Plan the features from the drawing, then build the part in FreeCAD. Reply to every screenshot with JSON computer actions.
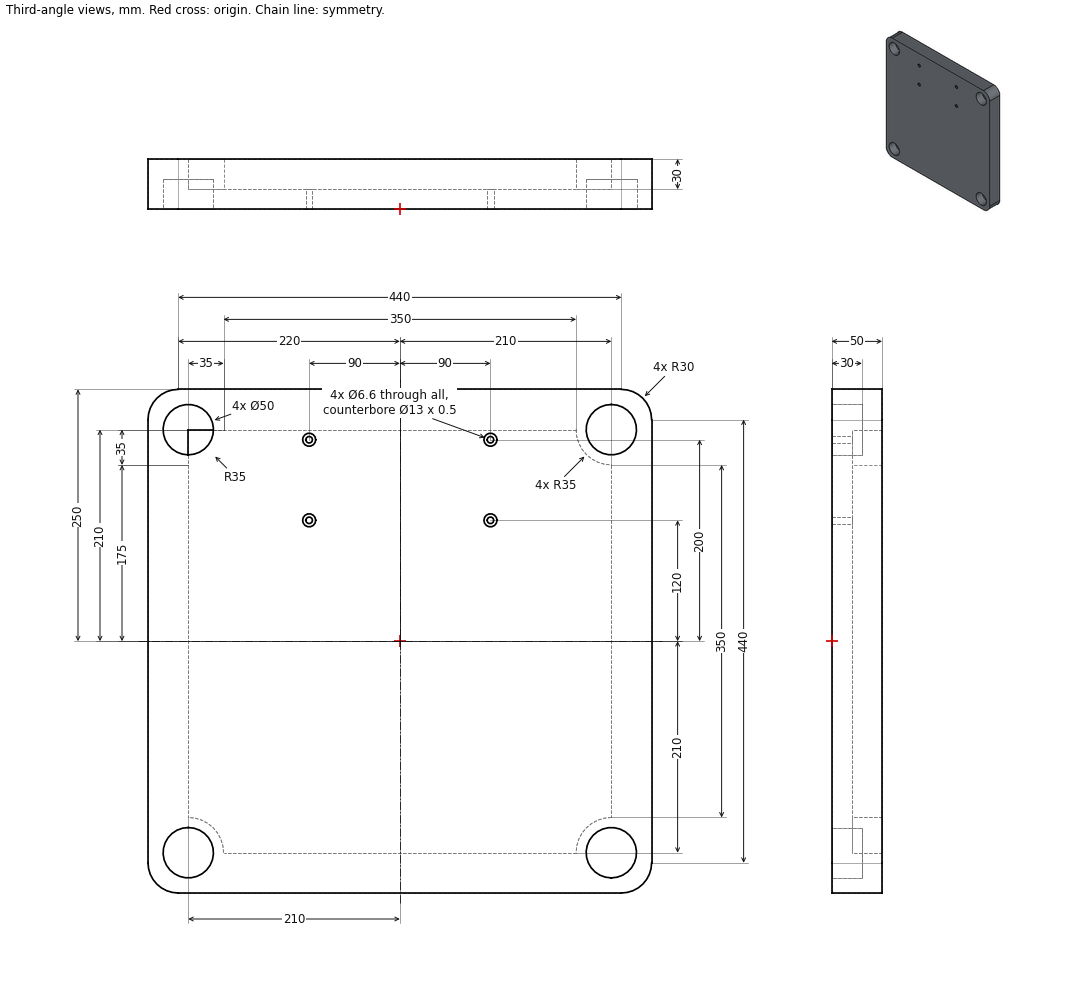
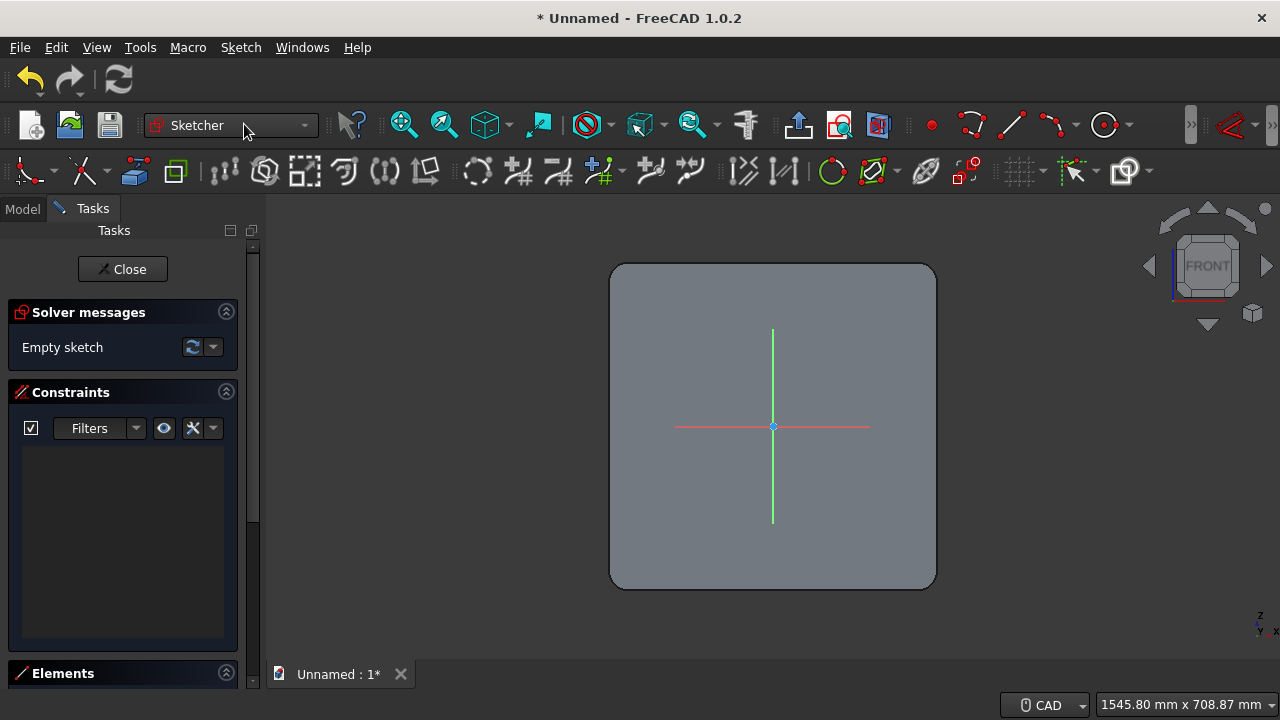
{"action": "key", "text": "g c"}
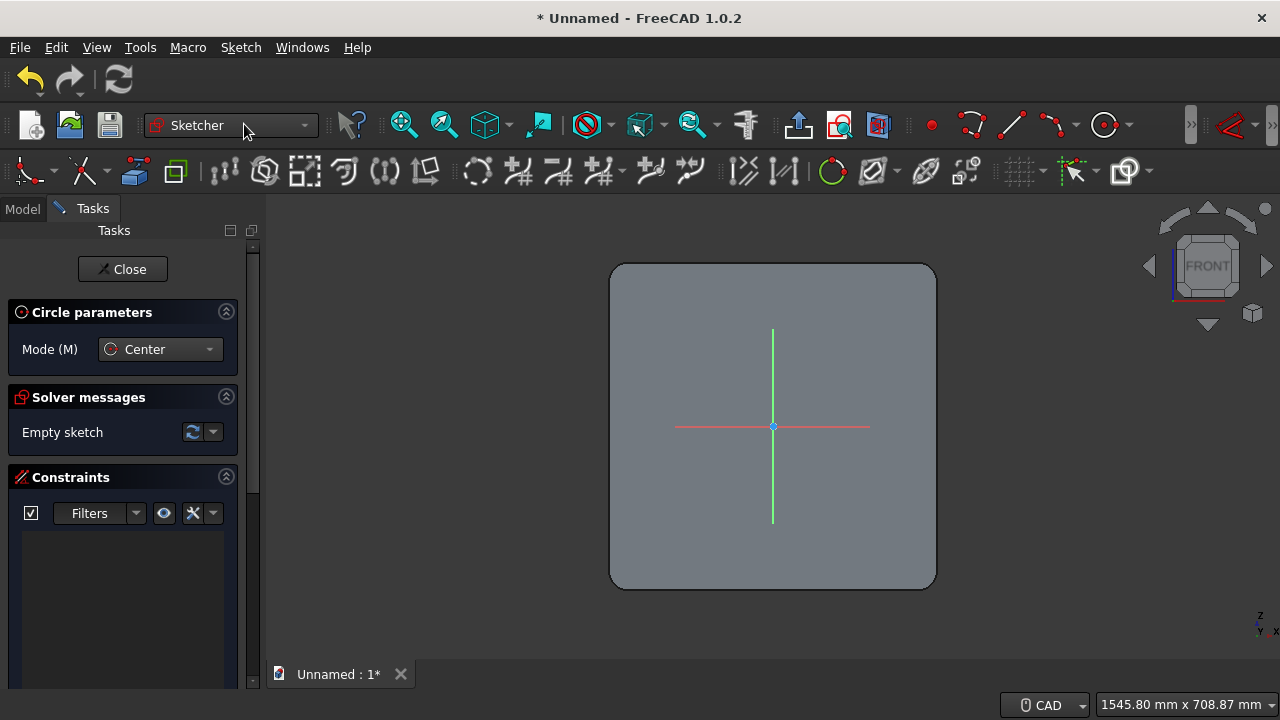
{"action": "scroll", "coordinate": [635, 289], "scroll_direction": "up", "scroll_amount": 2}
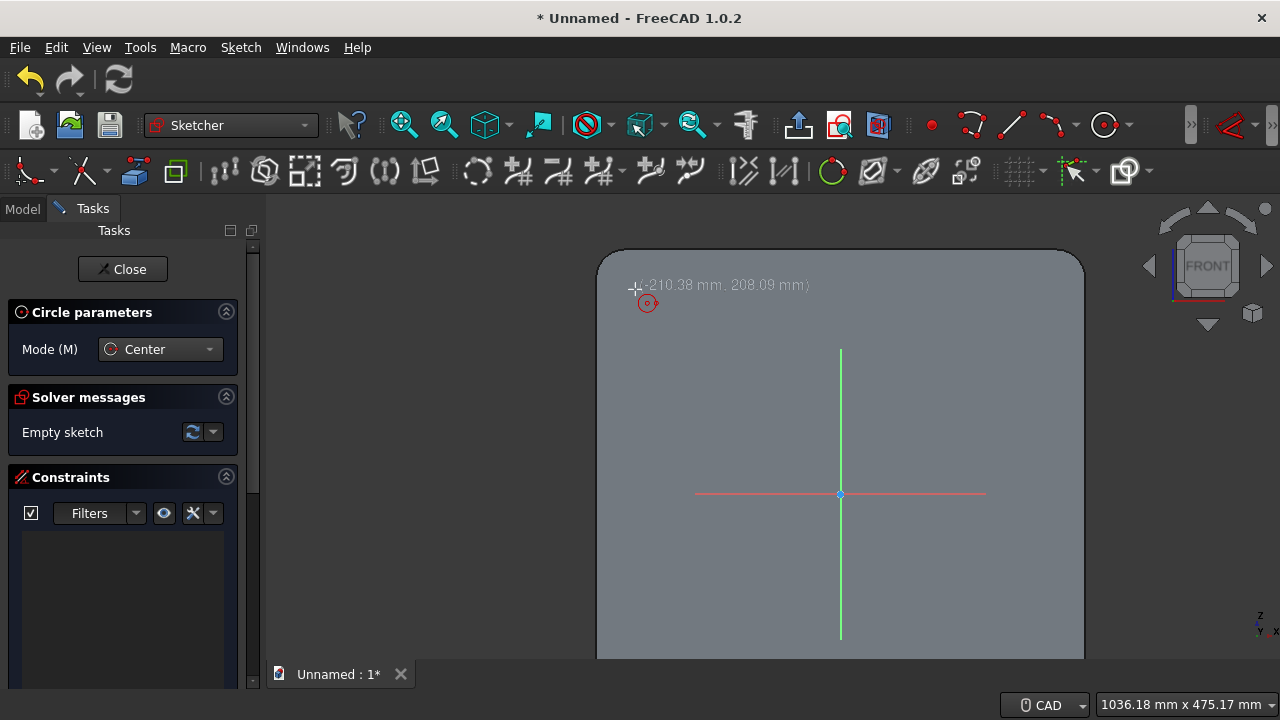
{"action": "left_click", "coordinate": [635, 289]}
{"action": "left_click", "coordinate": [652, 271]}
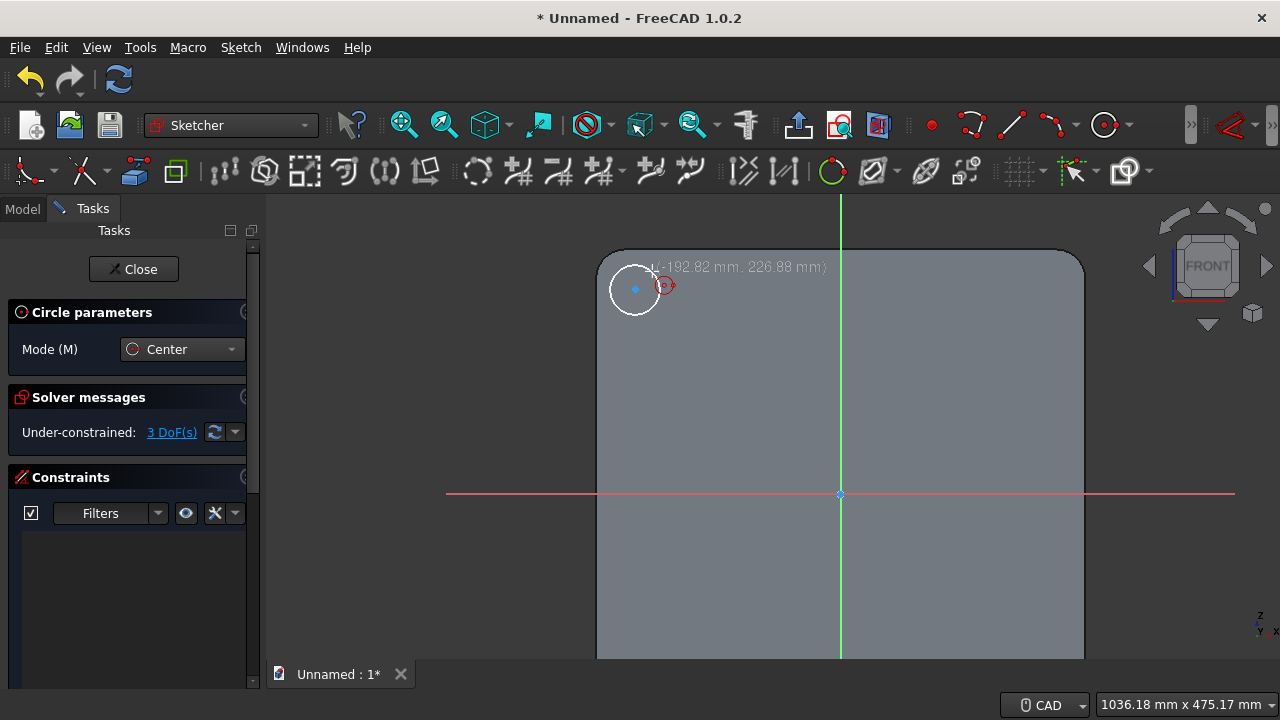
{"action": "left_click", "coordinate": [1046, 289]}
{"action": "left_click", "coordinate": [1063, 271]}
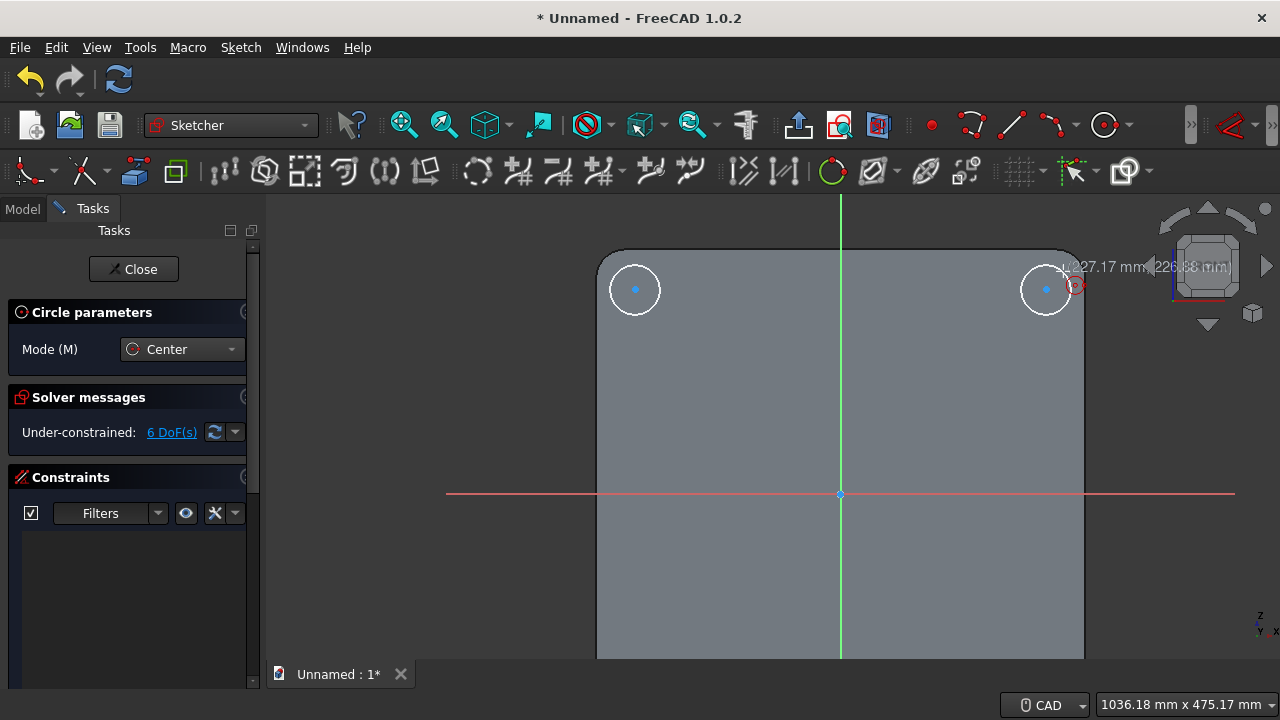
{"action": "scroll", "coordinate": [428, 289], "scroll_direction": "down", "scroll_amount": 2}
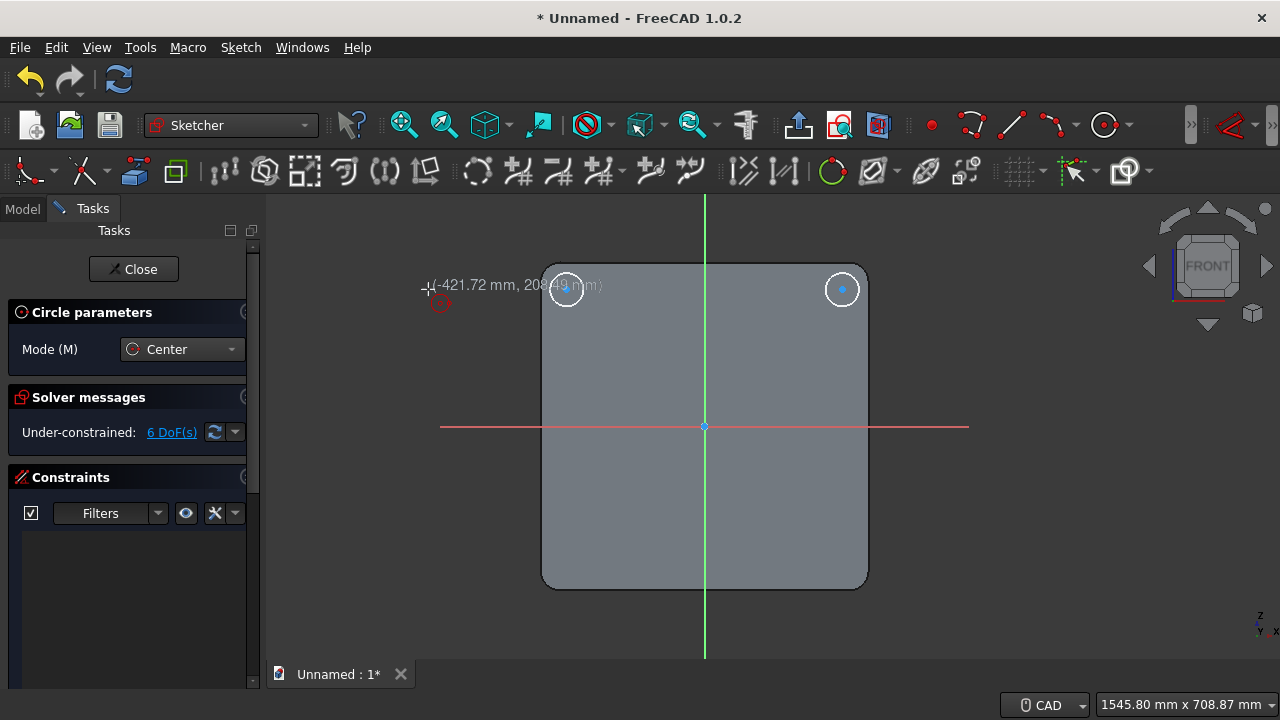
{"action": "scroll", "coordinate": [842, 564], "scroll_direction": "up", "scroll_amount": 2}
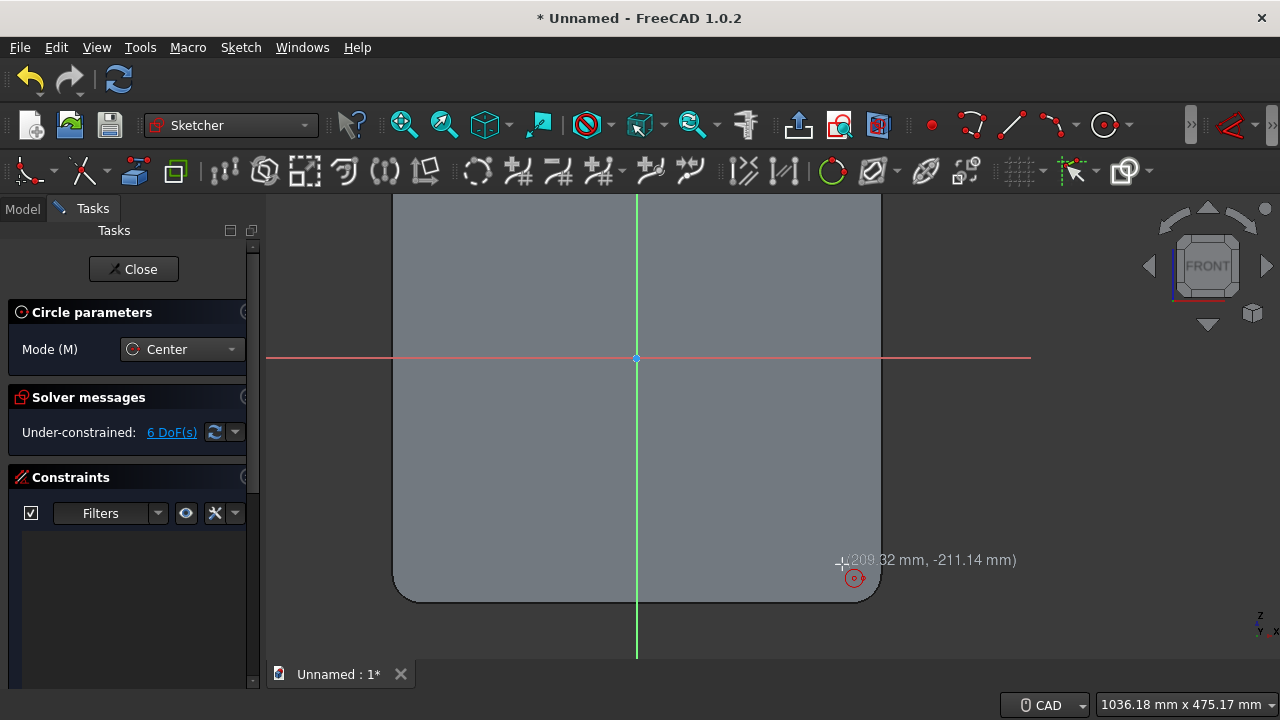
{"action": "left_click", "coordinate": [842, 564]}
{"action": "left_click", "coordinate": [860, 547]}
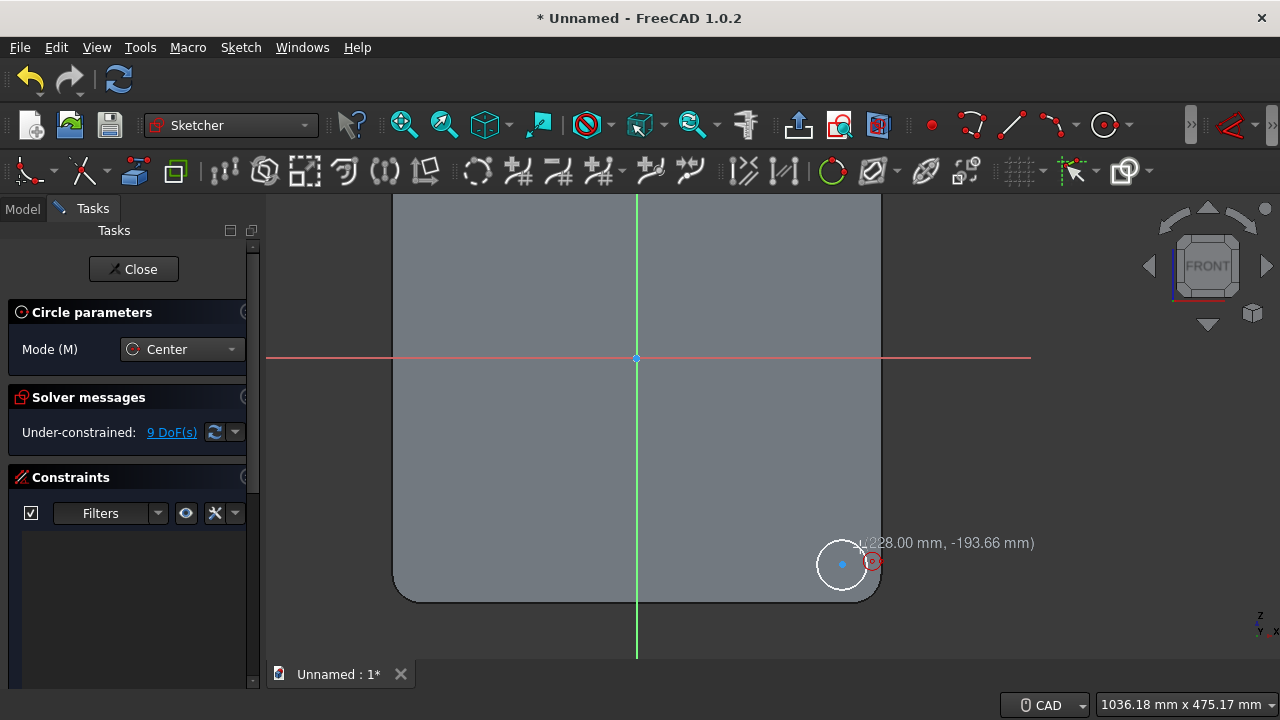
{"action": "left_click", "coordinate": [431, 564]}
{"action": "left_click", "coordinate": [449, 547]}
{"action": "key", "text": "Escape"}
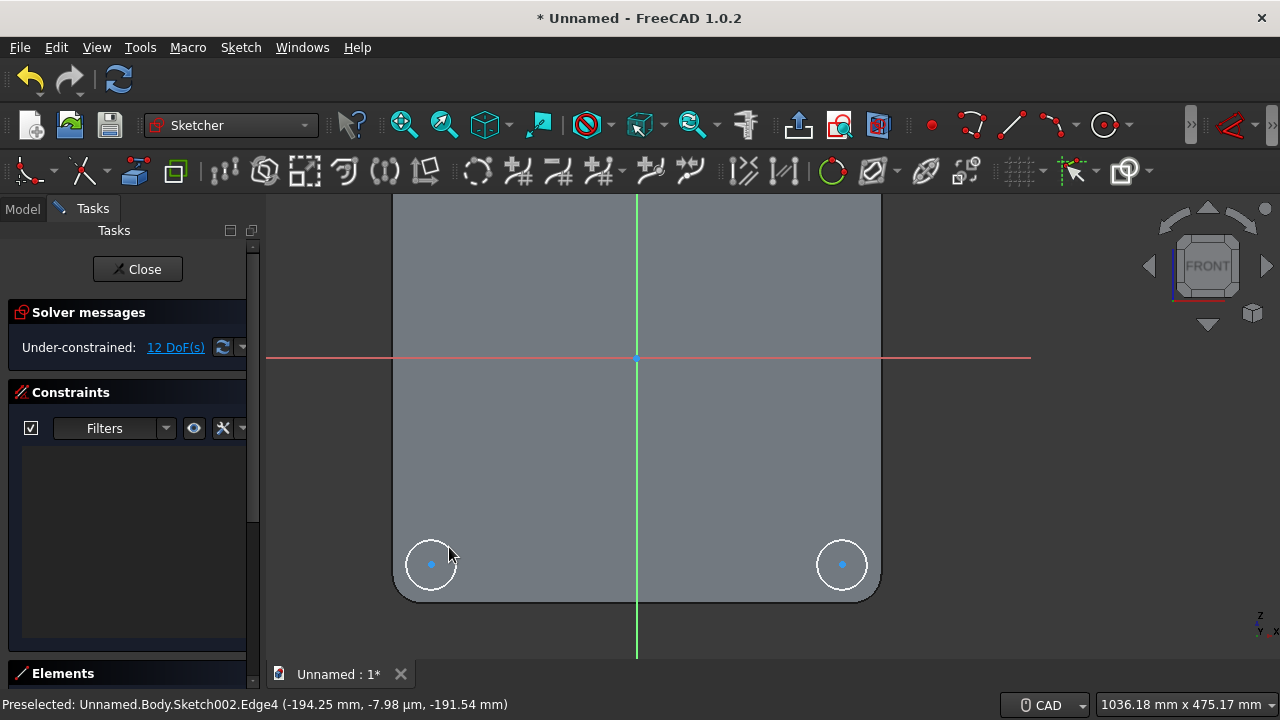
{"action": "scroll", "coordinate": [842, 565], "scroll_direction": "down", "scroll_amount": 2}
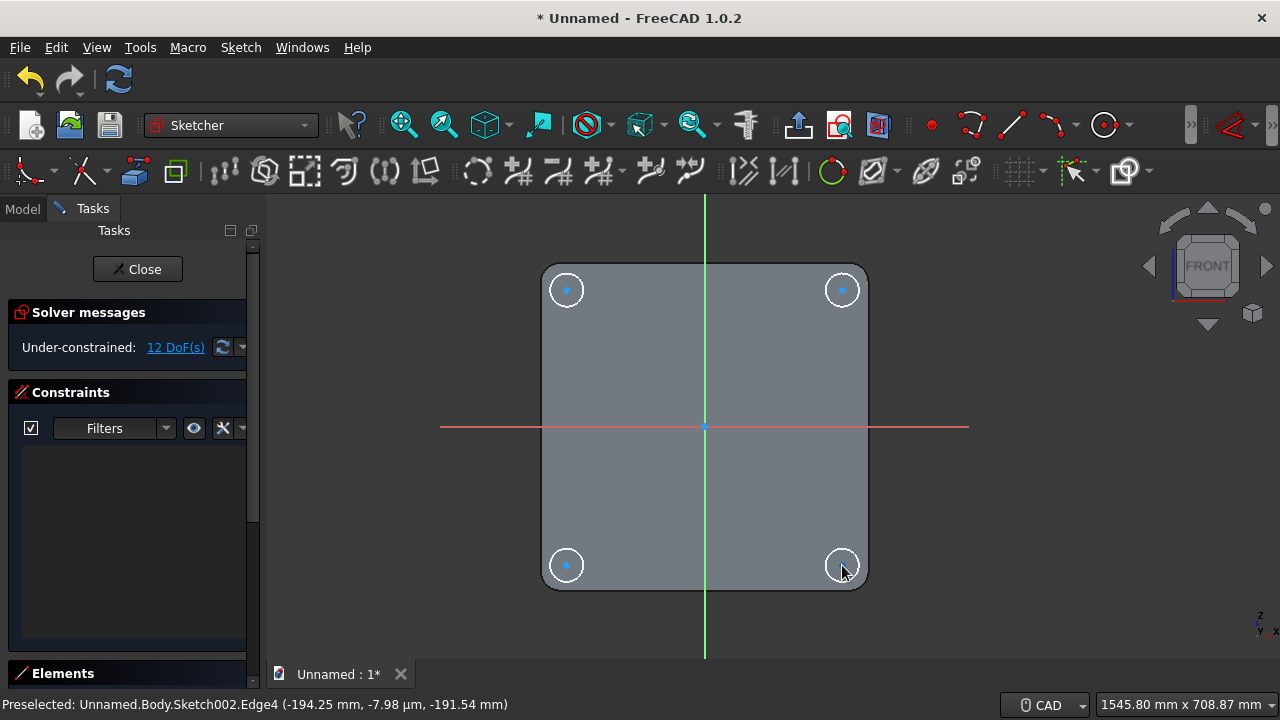
{"action": "left_click", "coordinate": [579, 278]}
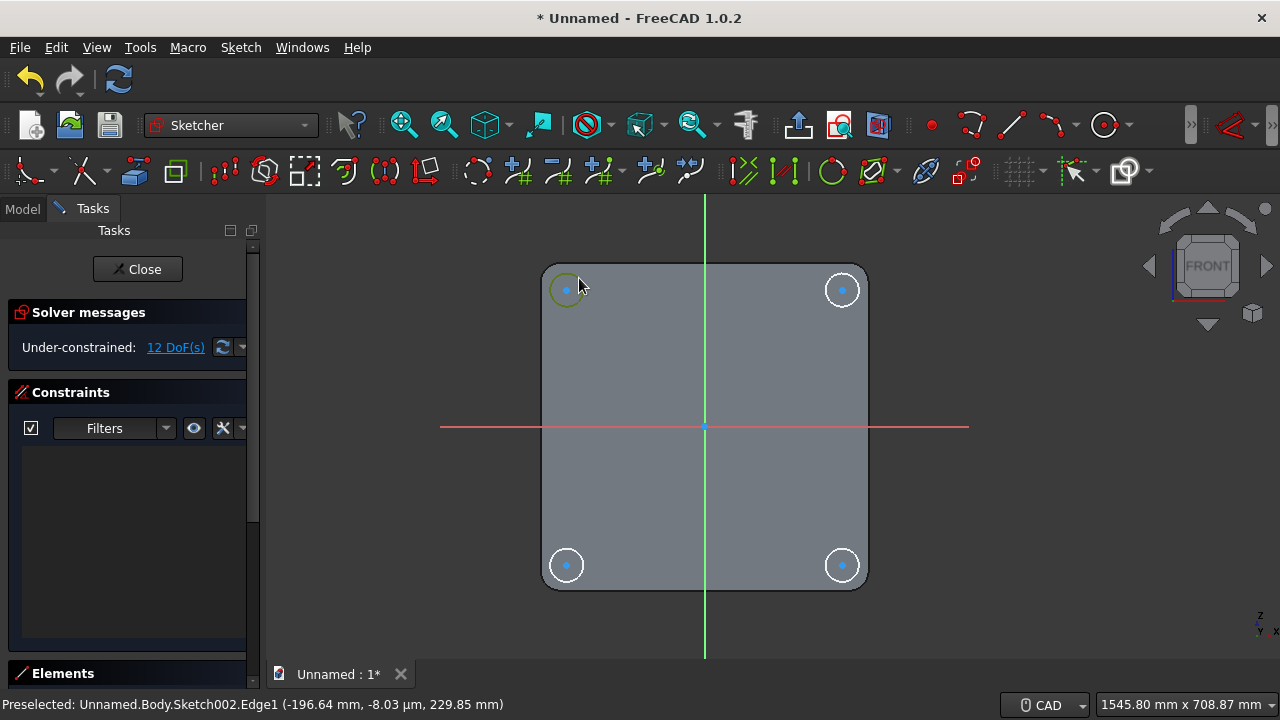
{"action": "left_click", "coordinate": [854, 278]}